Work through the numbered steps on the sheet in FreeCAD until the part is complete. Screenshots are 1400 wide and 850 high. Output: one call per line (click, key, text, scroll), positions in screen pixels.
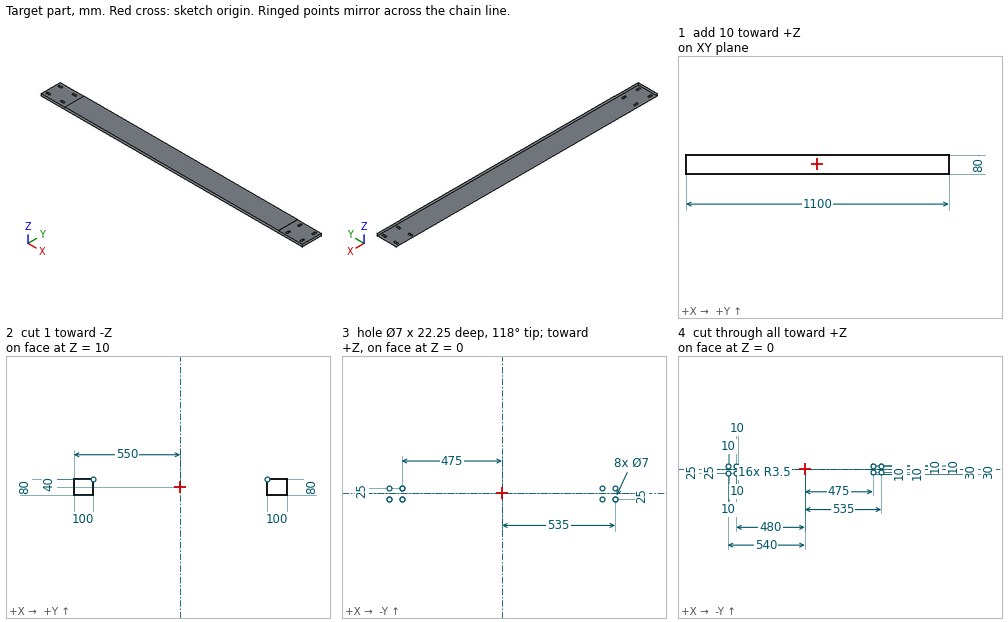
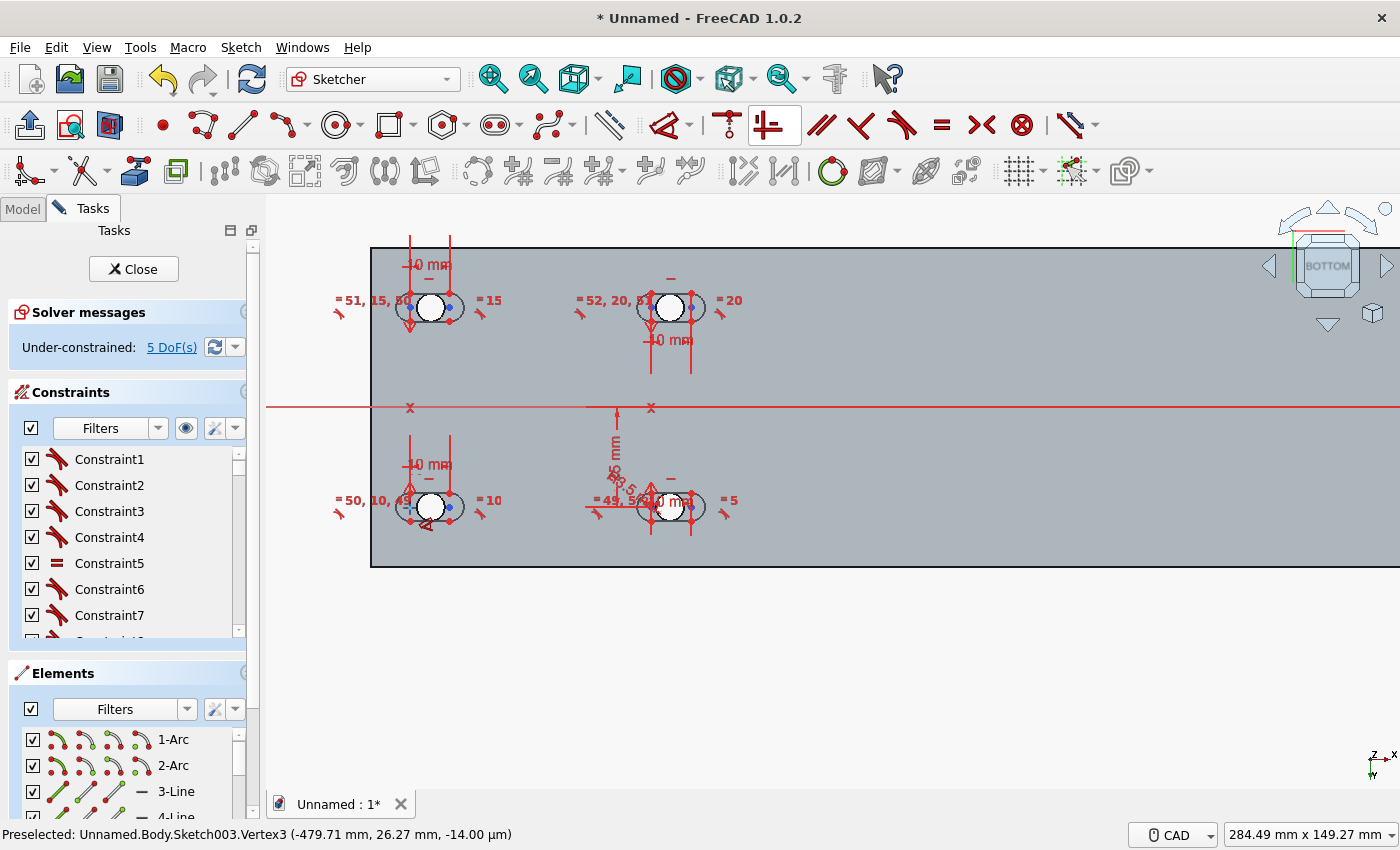
click(410, 507)
click(376, 434)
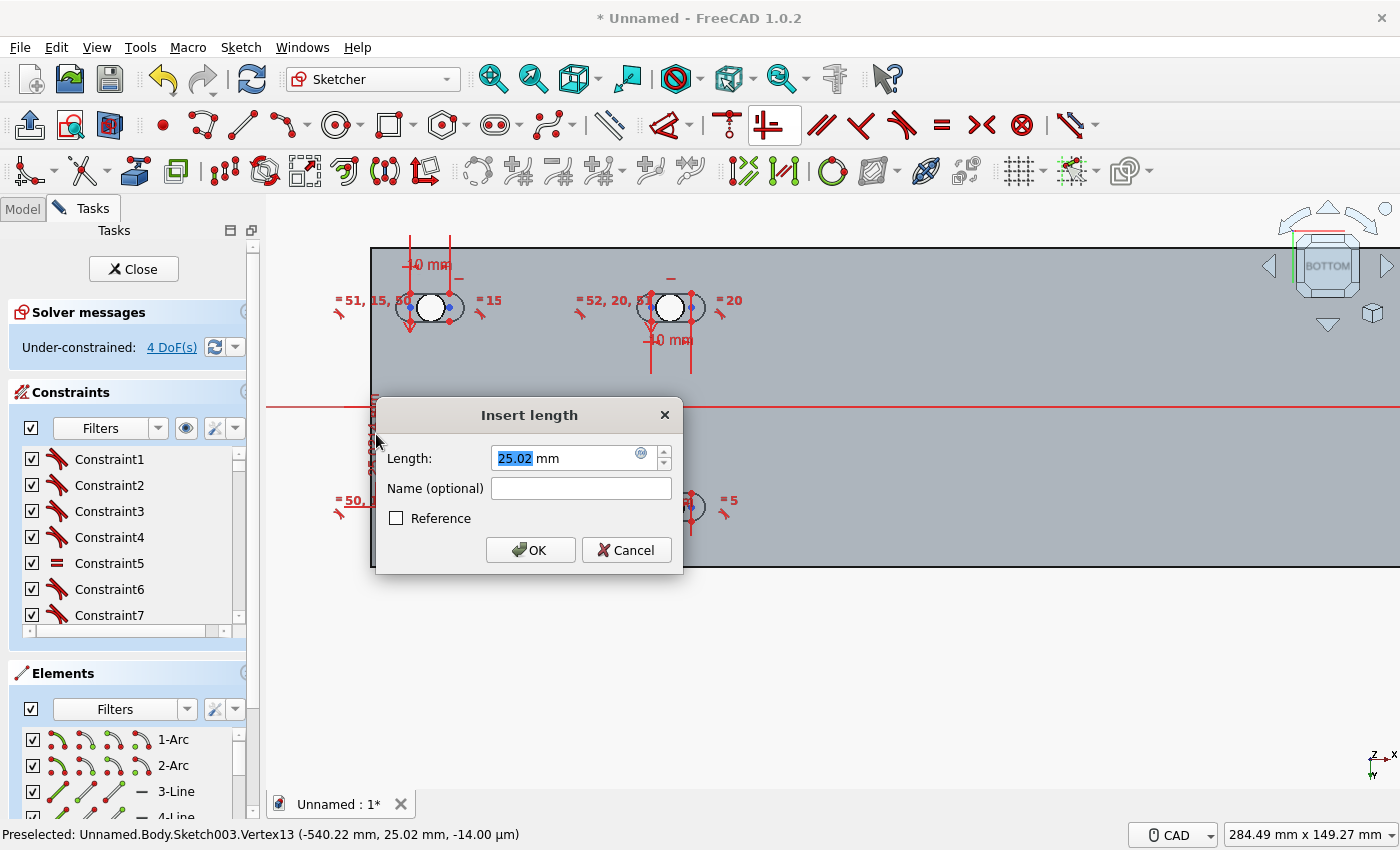
text(25)
key(Return)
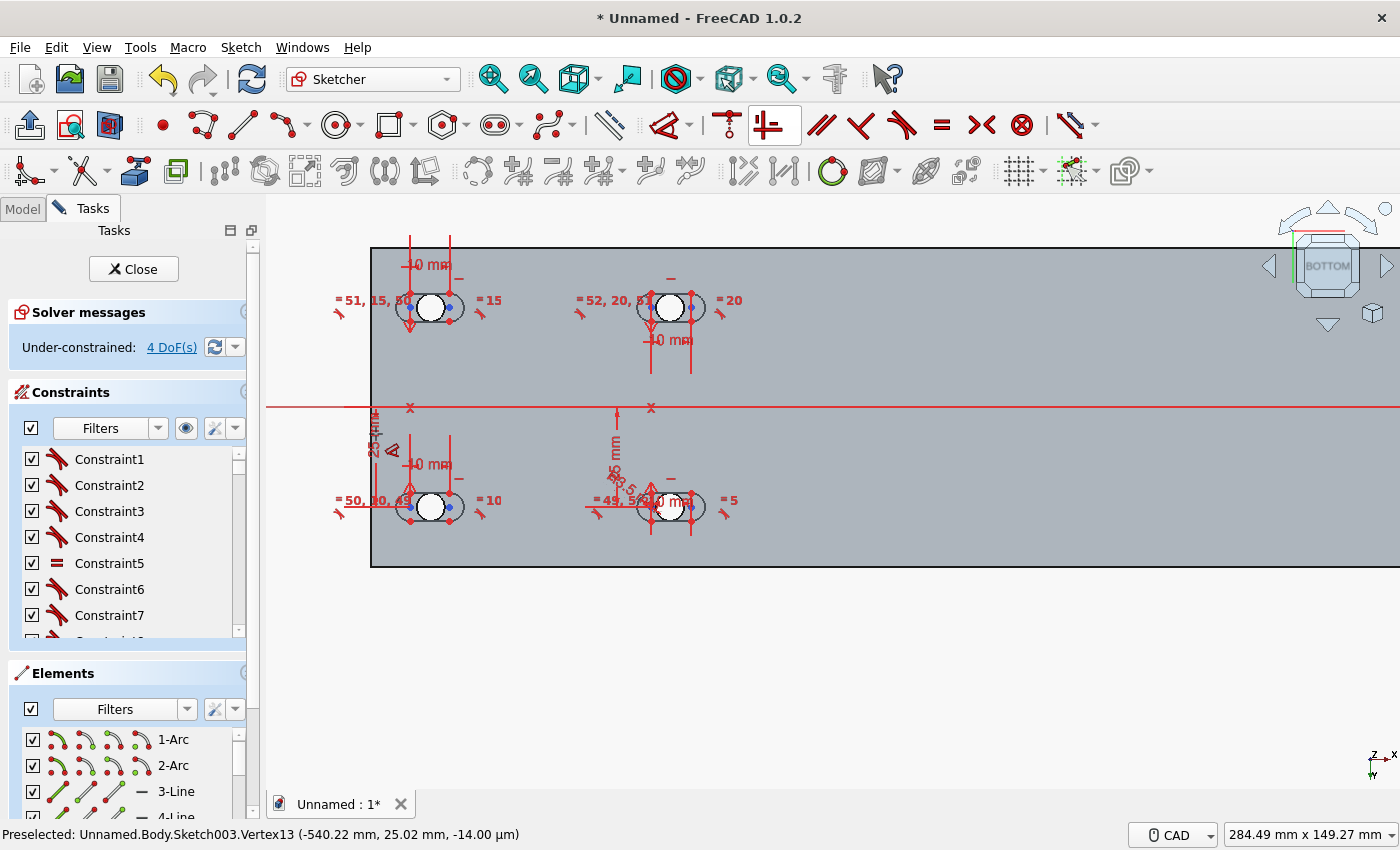
click(651, 493)
click(943, 527)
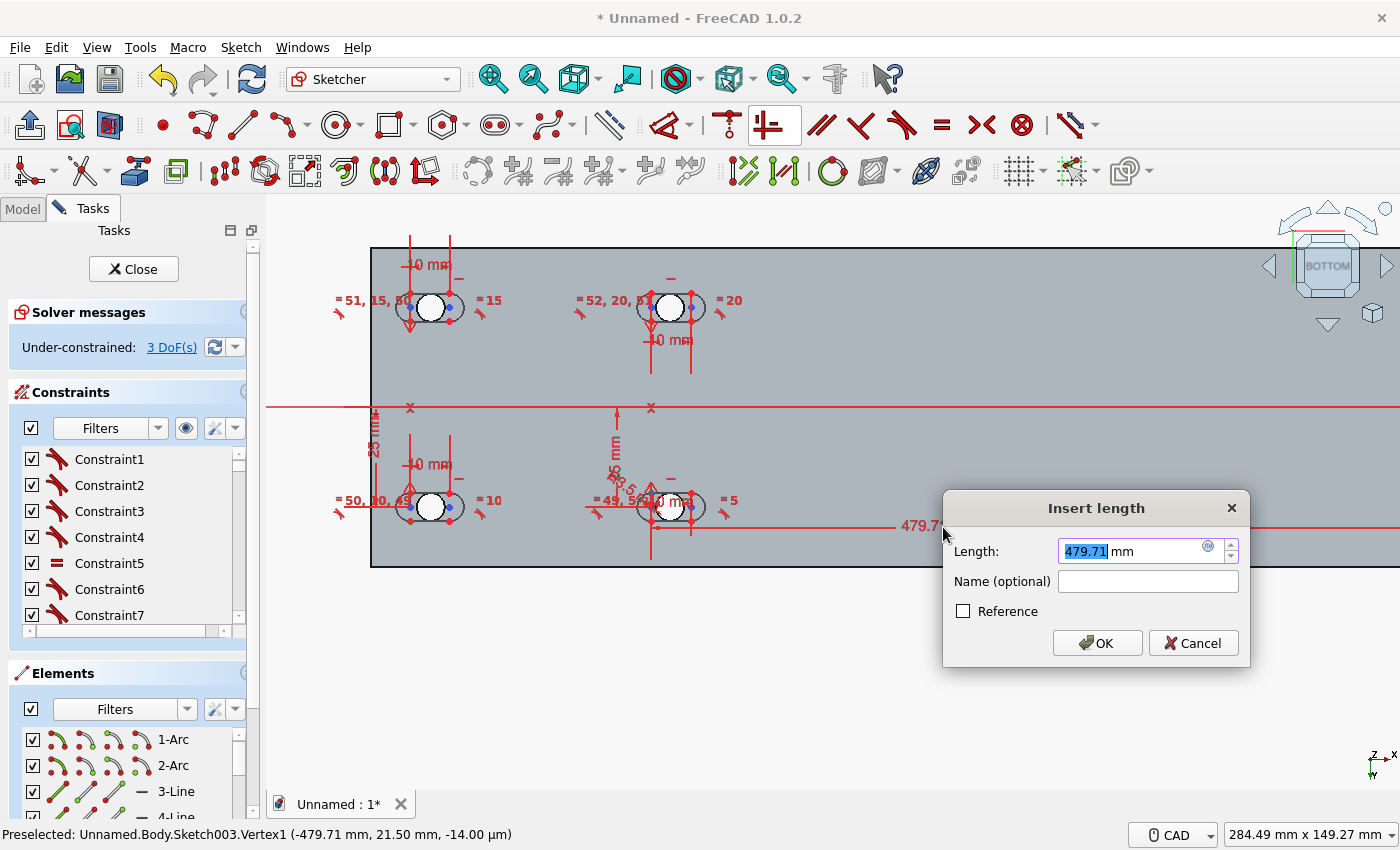
text(480)
key(Return)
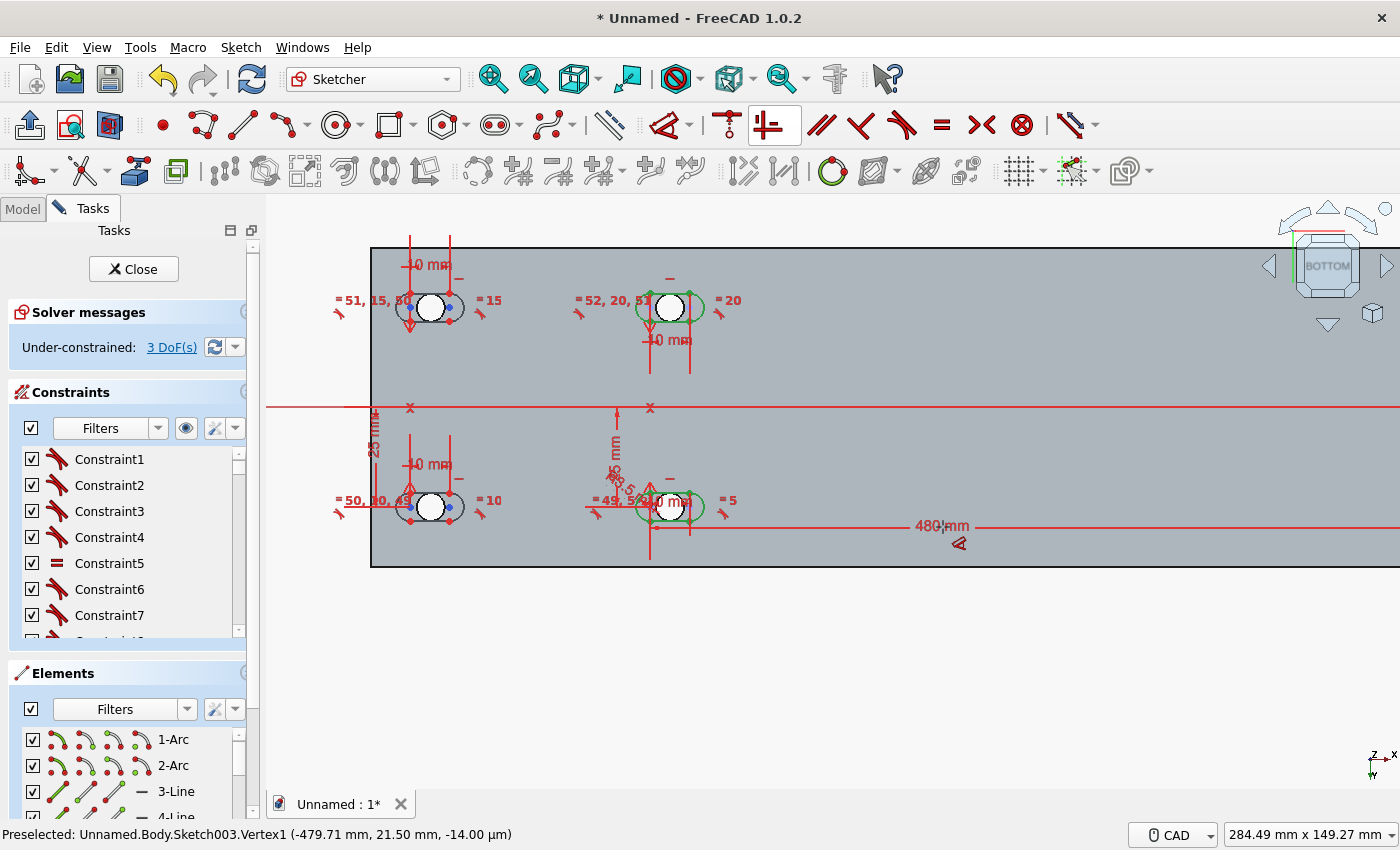
click(410, 493)
click(823, 527)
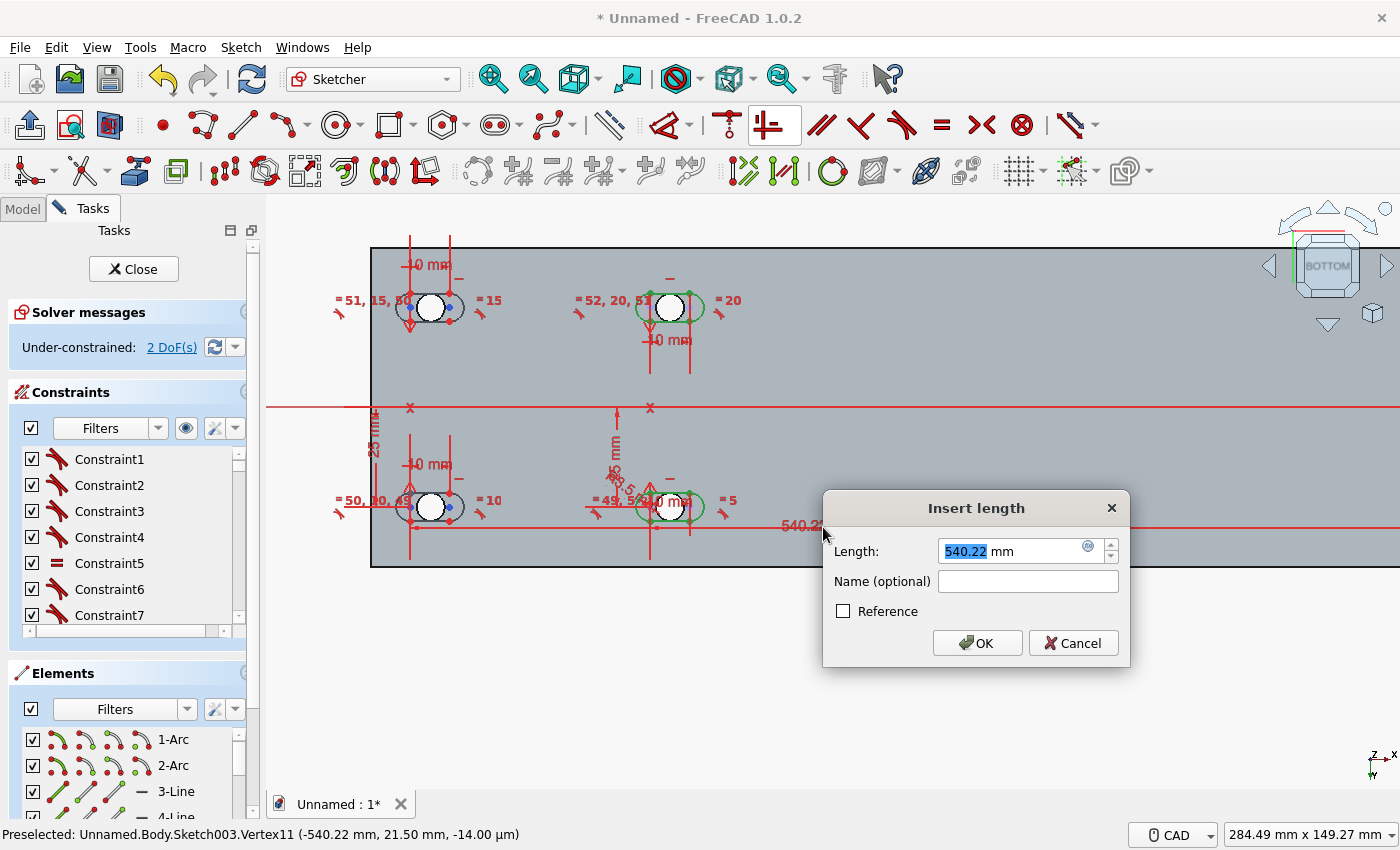
text(540)
key(Return)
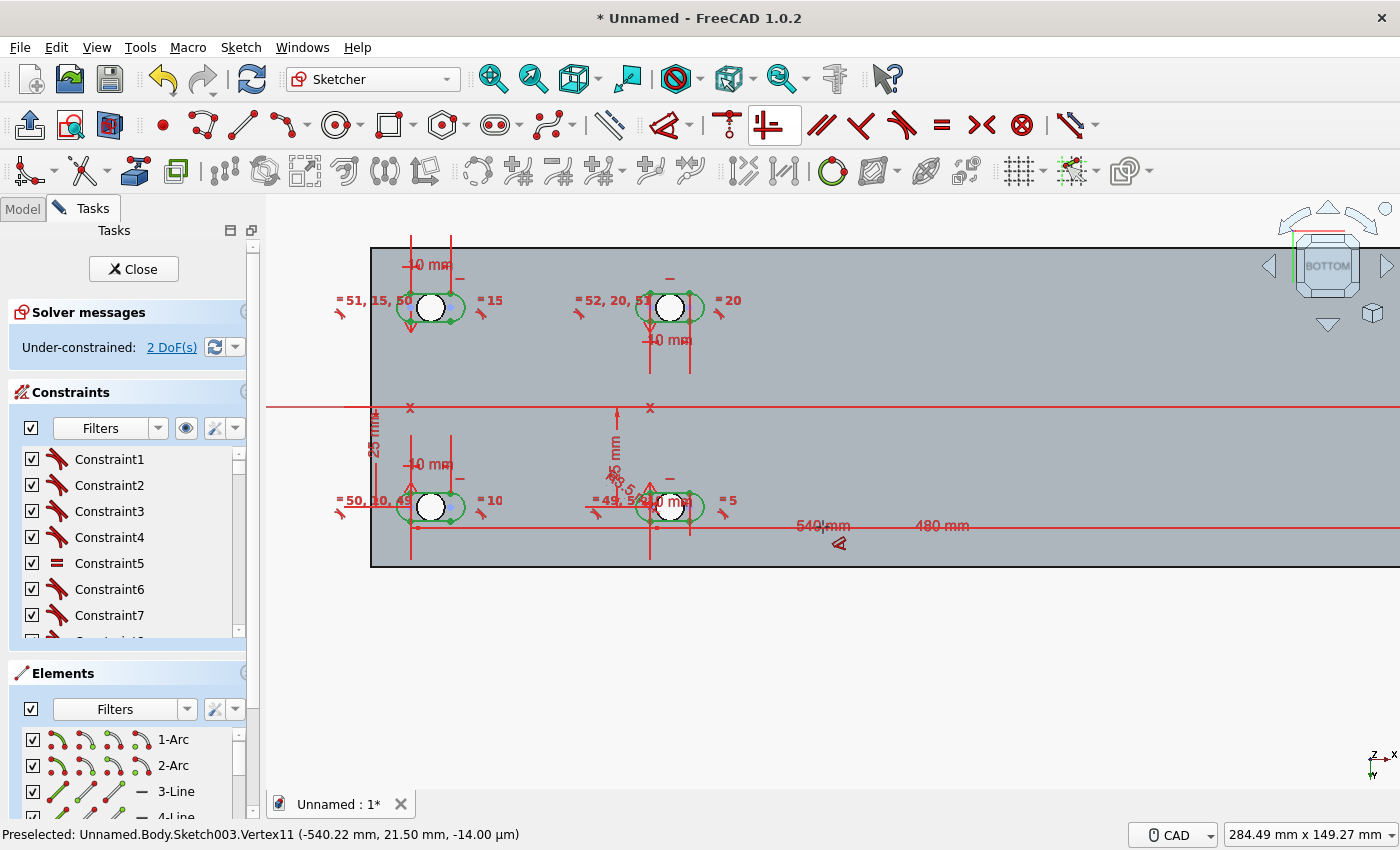
scroll(410, 508, down, 9)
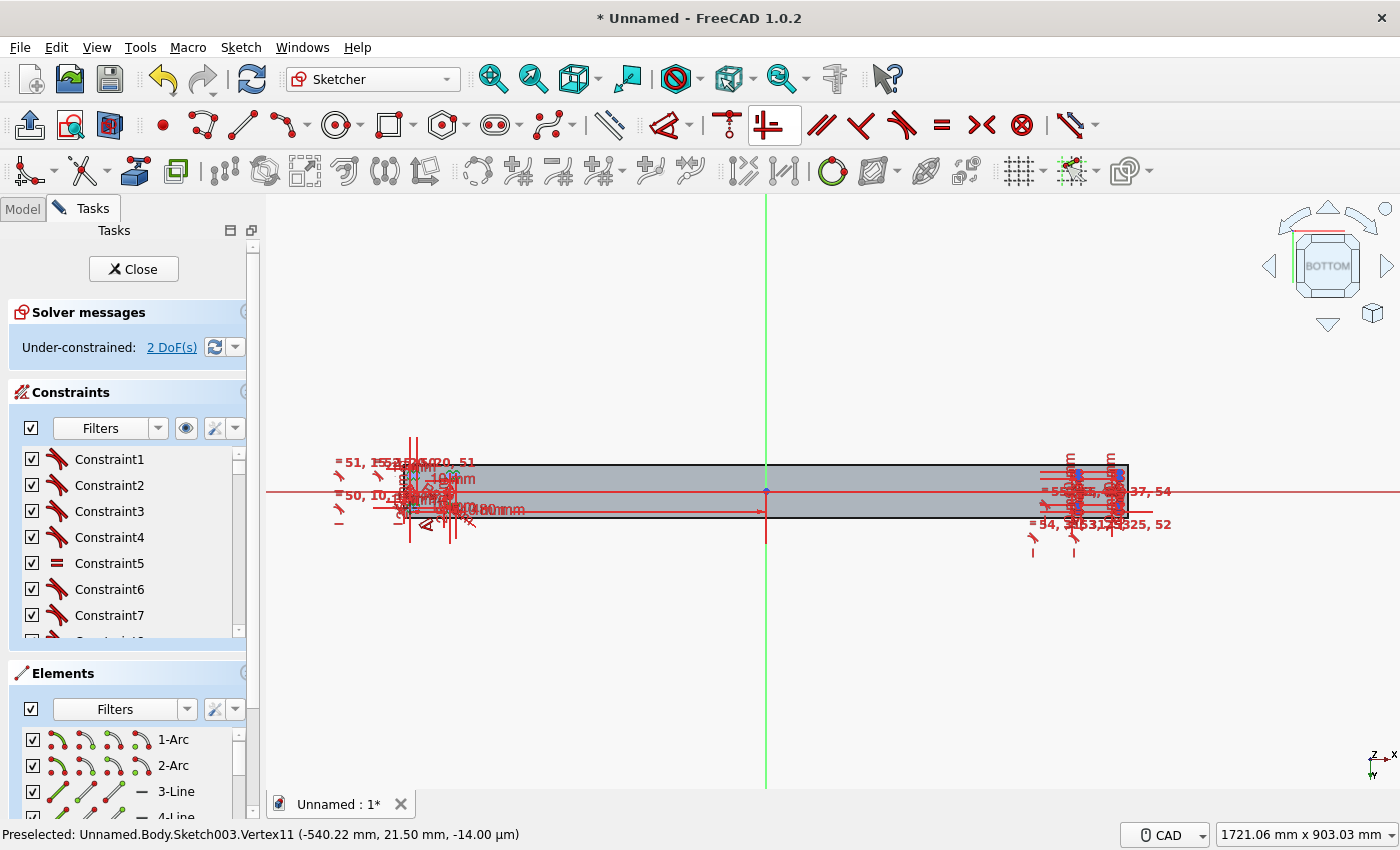
scroll(1119, 512, up, 9)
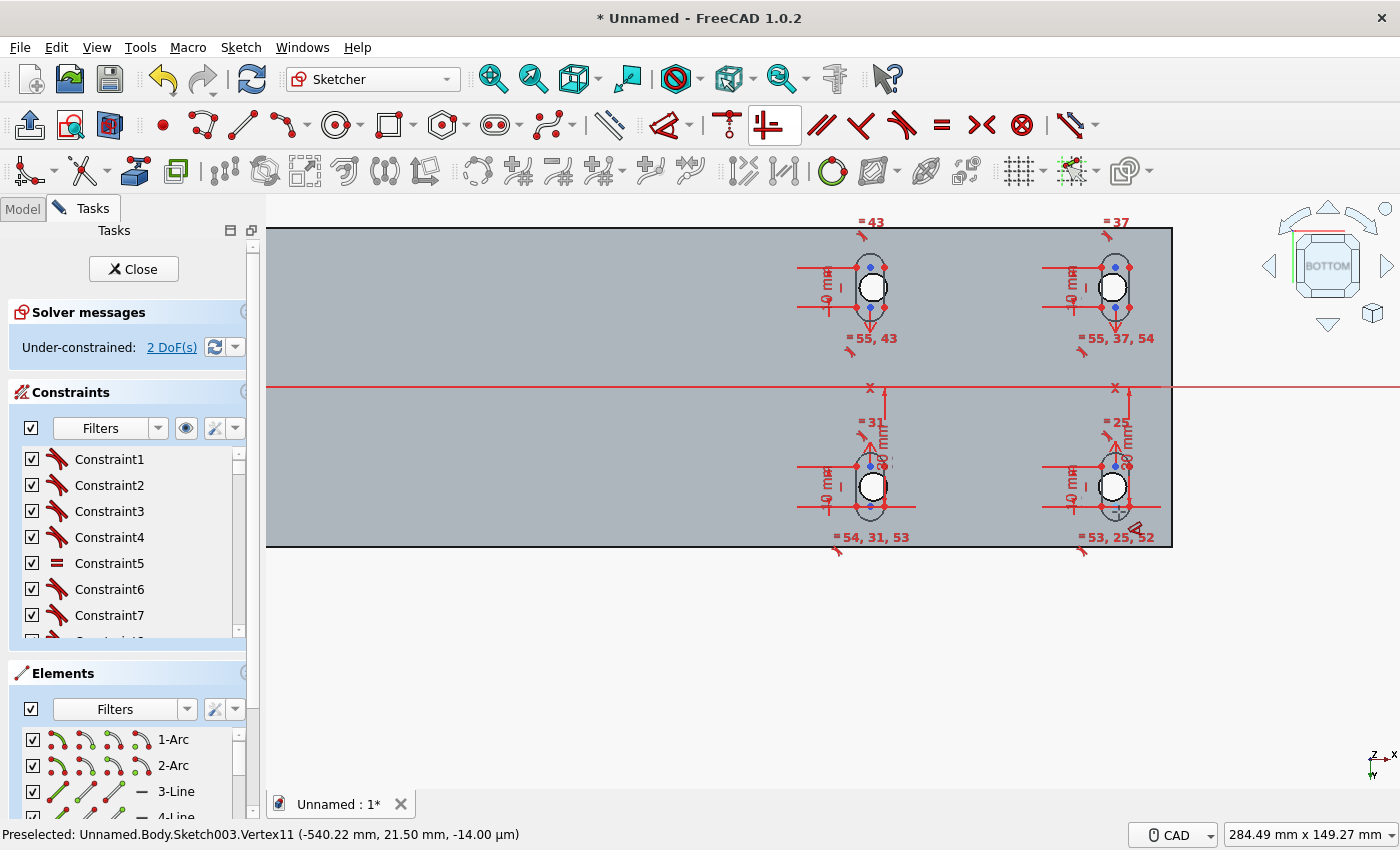
click(1116, 507)
click(705, 541)